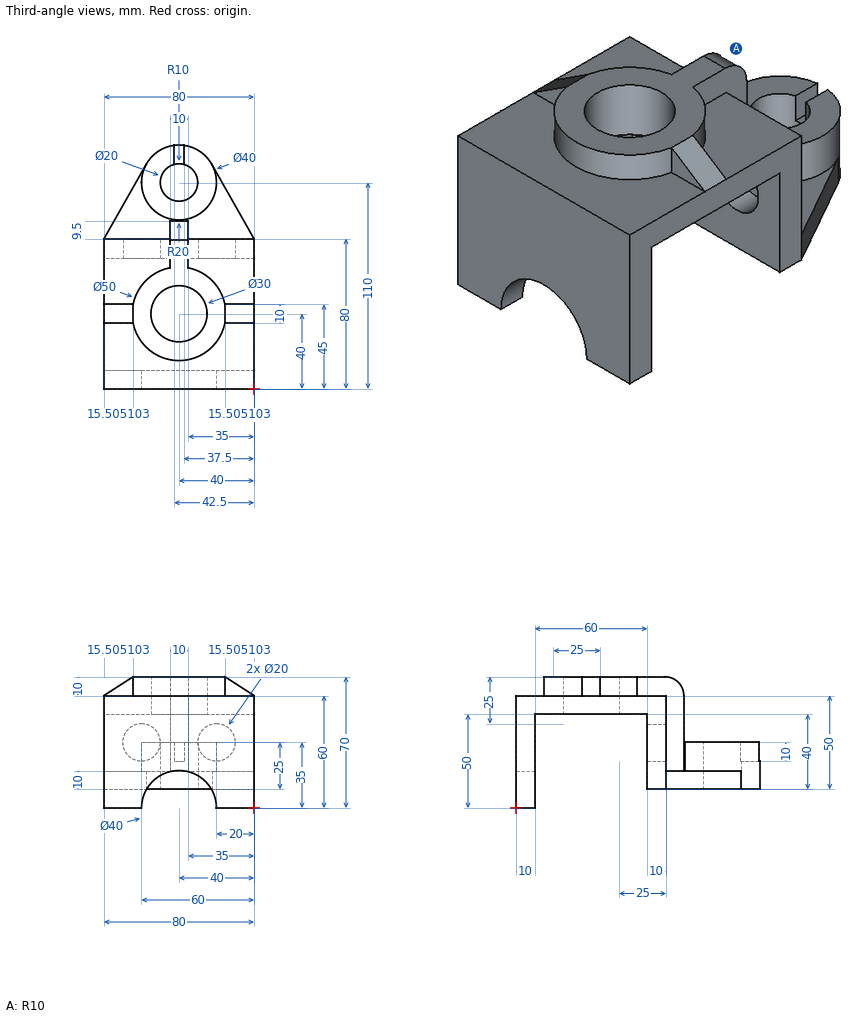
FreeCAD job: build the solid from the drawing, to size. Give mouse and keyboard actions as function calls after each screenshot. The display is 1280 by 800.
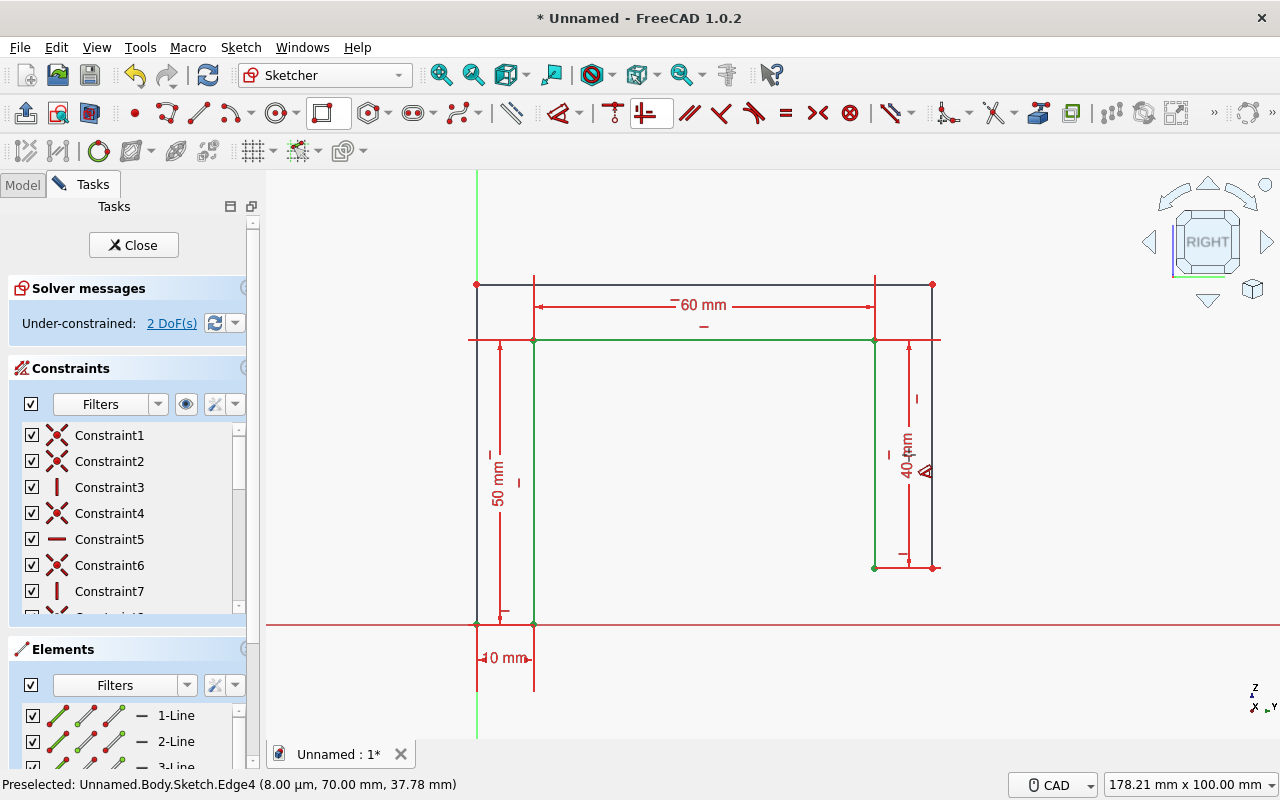
click(892, 568)
click(903, 602)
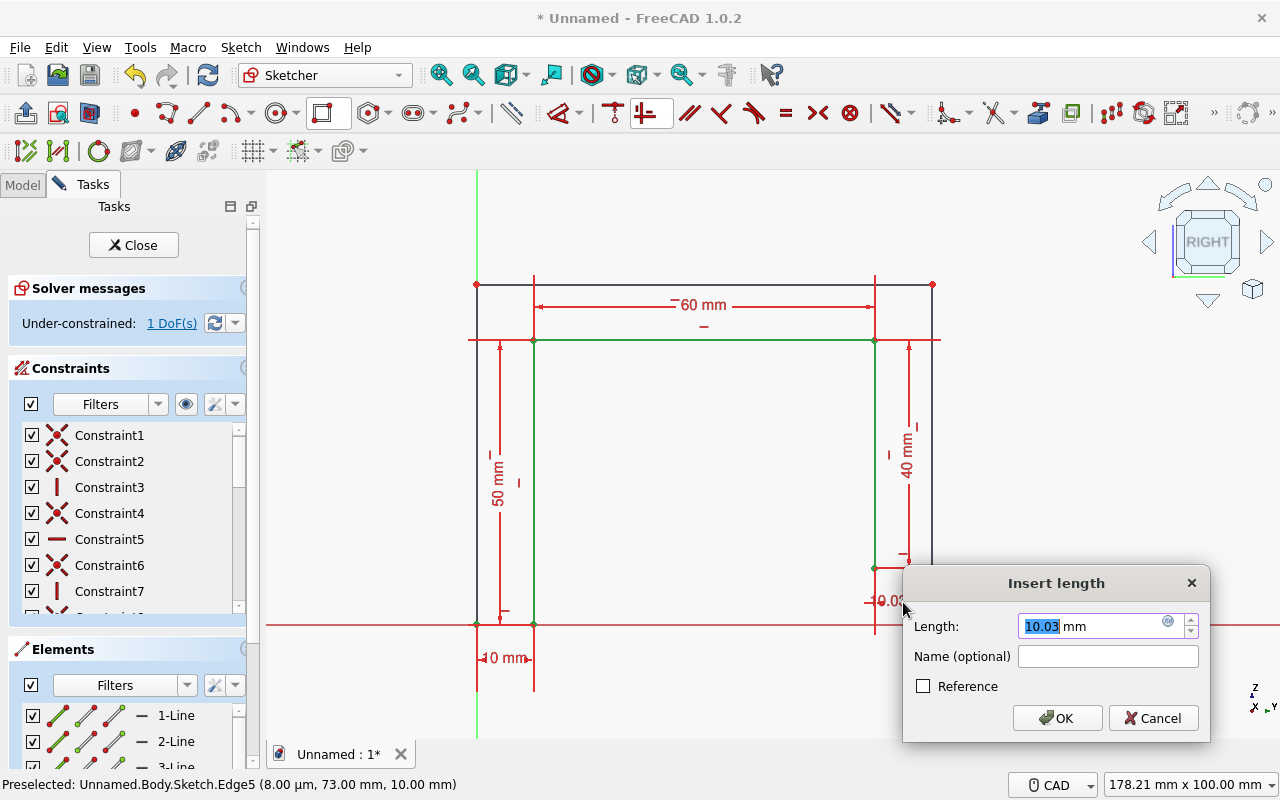
text(10)
key(Return)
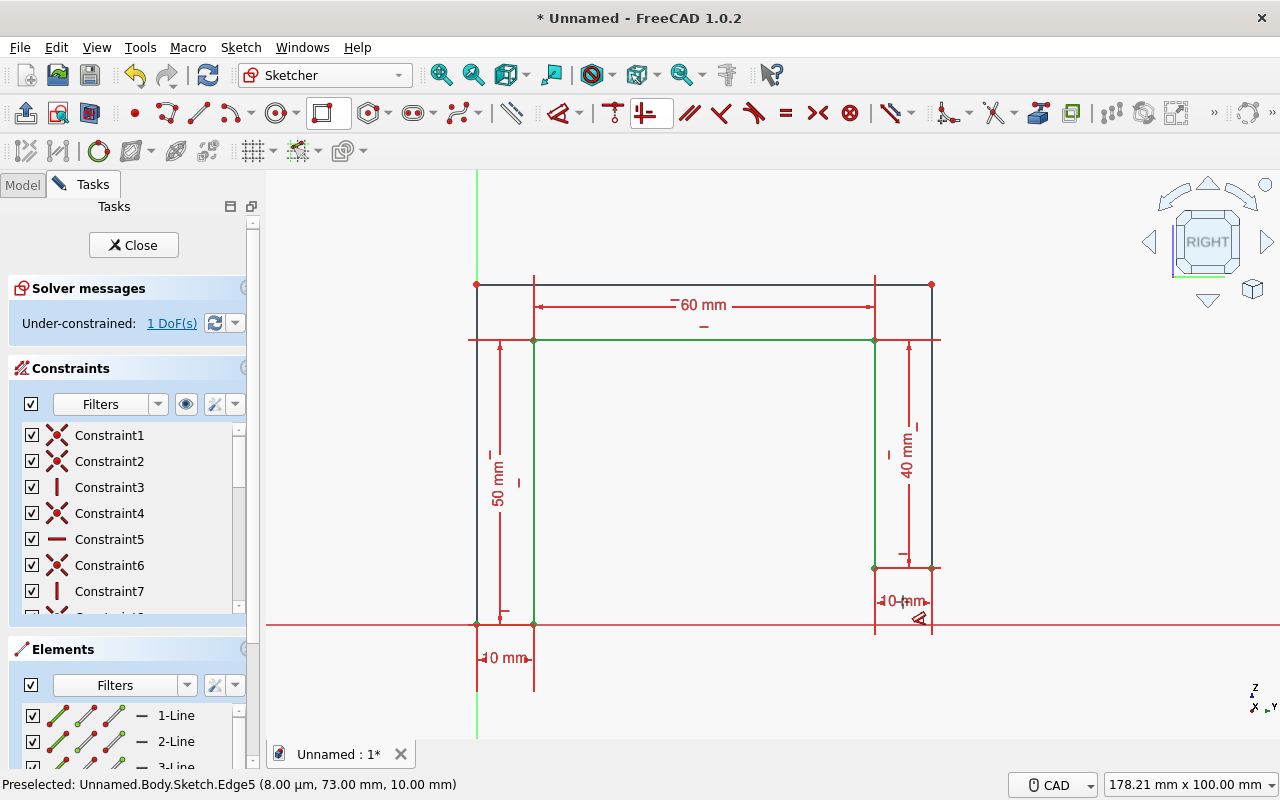
click(932, 483)
click(966, 427)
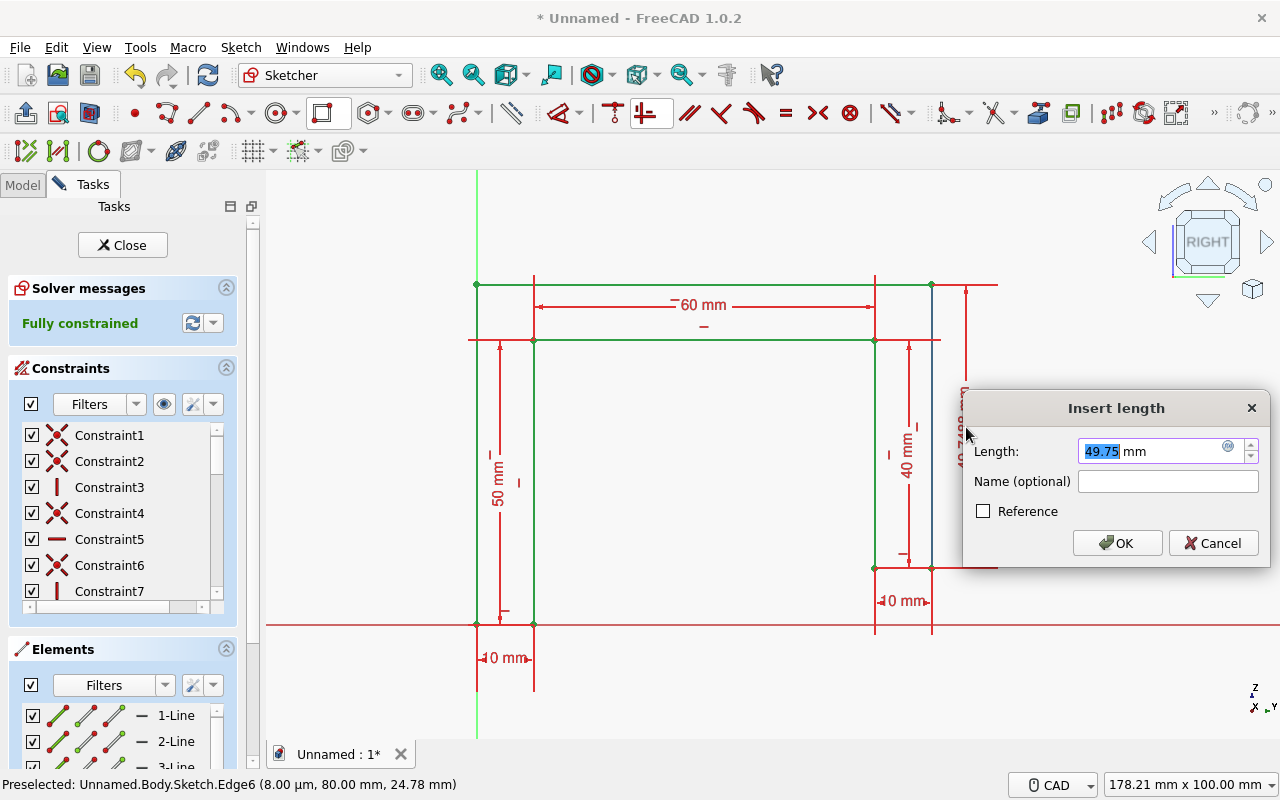
text(50)
key(Return)
key(Escape)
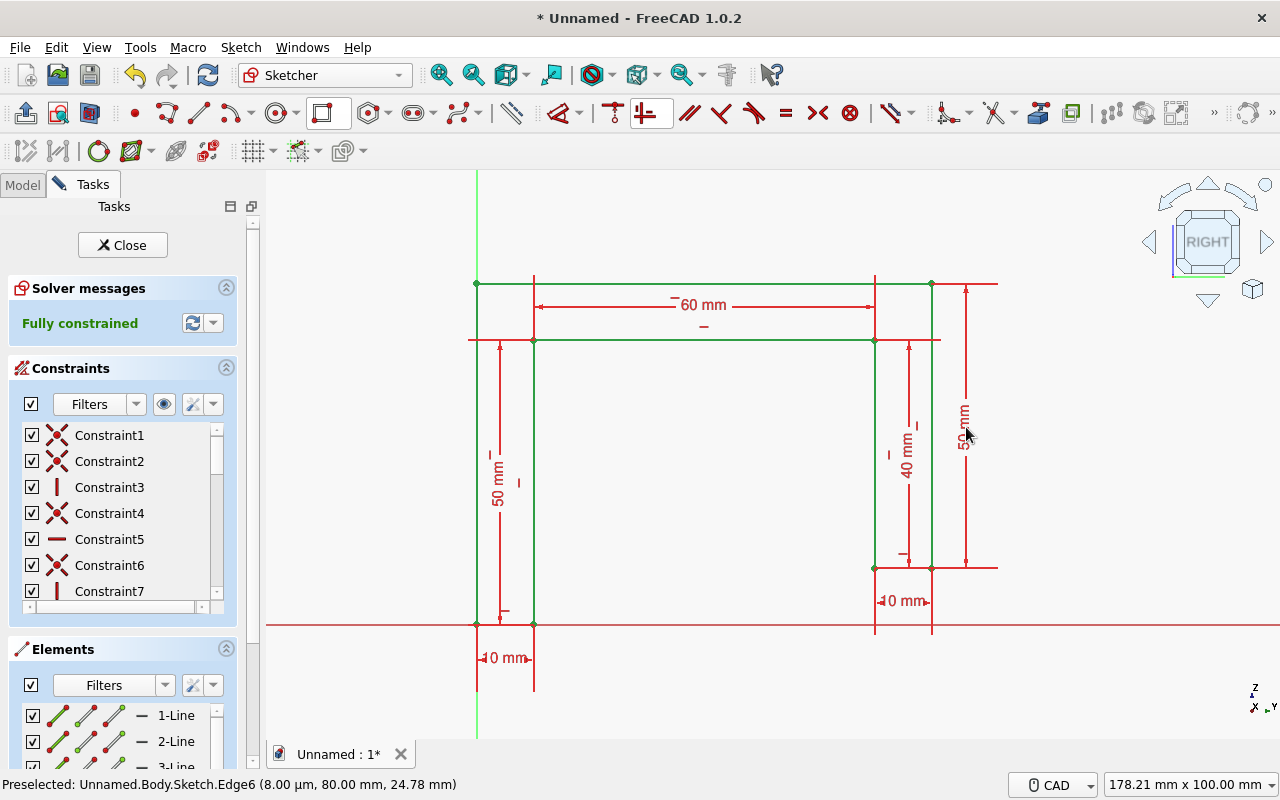
click(123, 245)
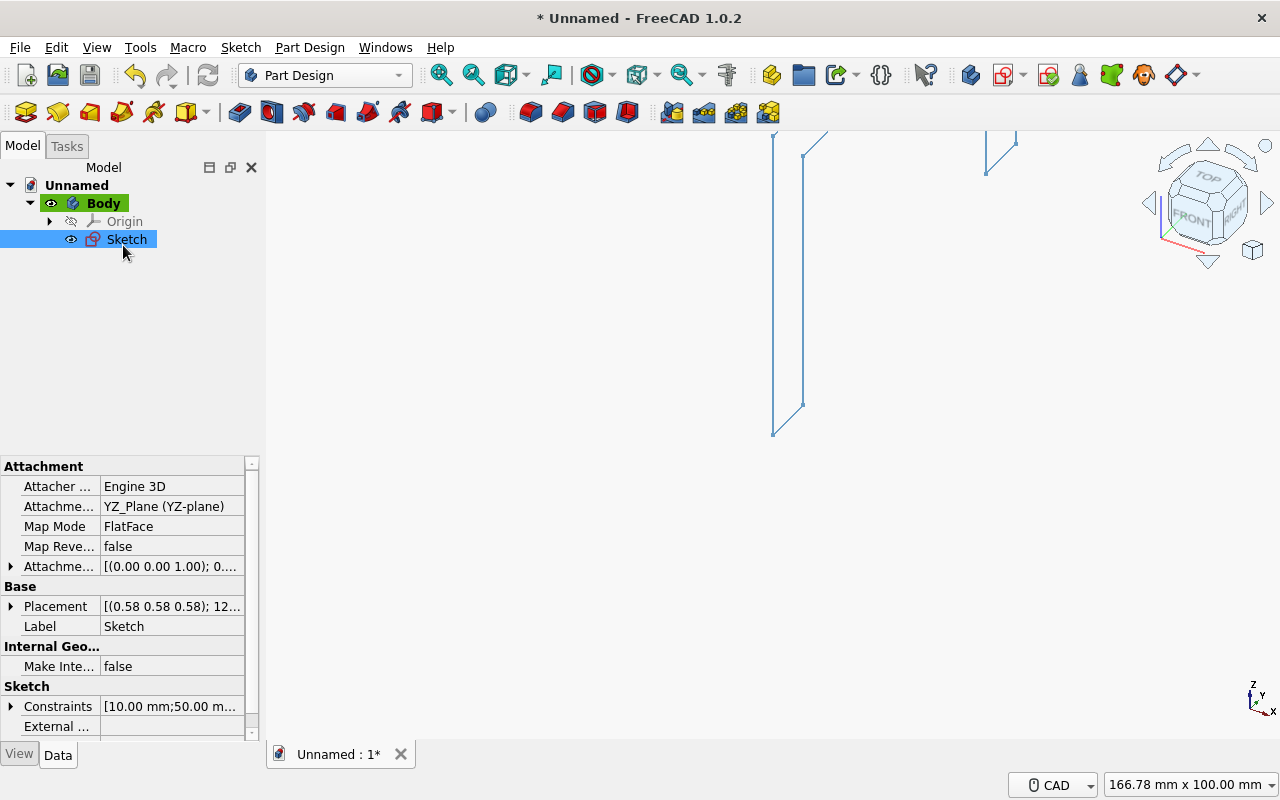
click(26, 112)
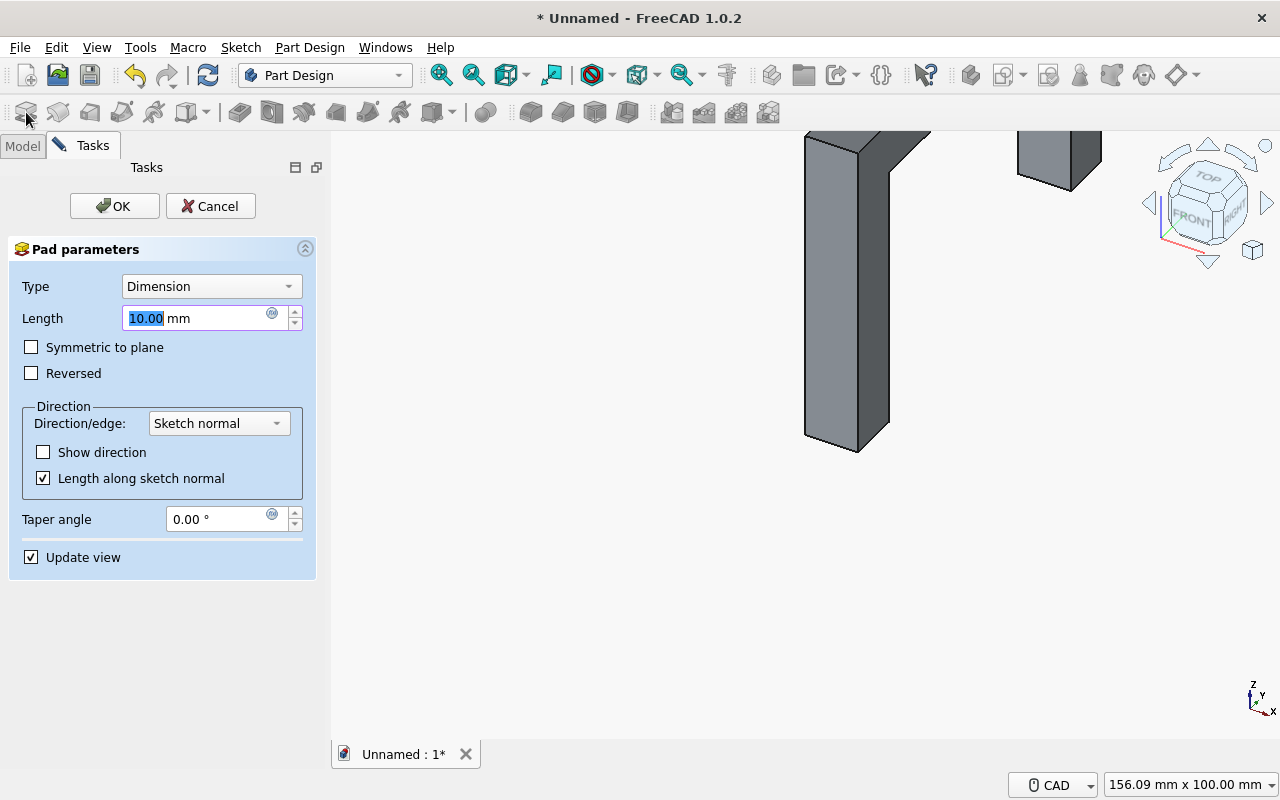
text(80)
key(Tab)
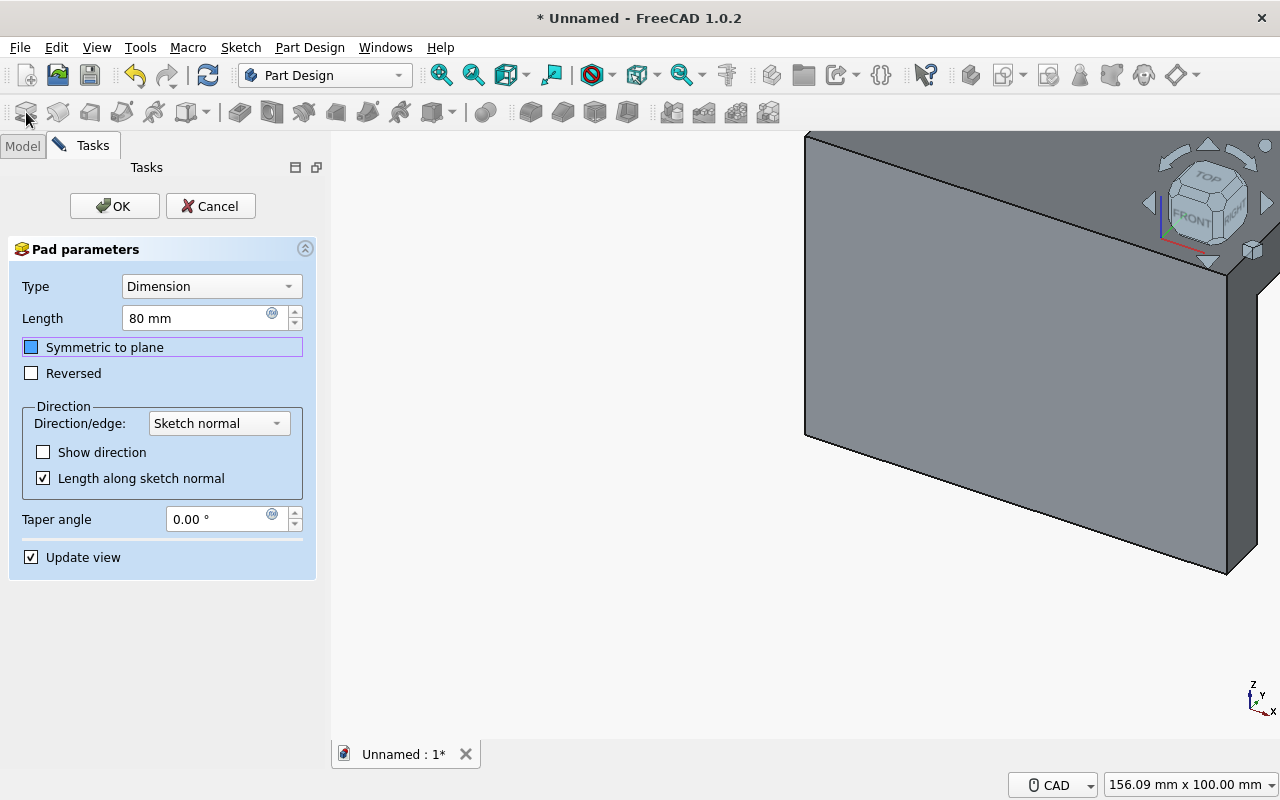
click(30, 373)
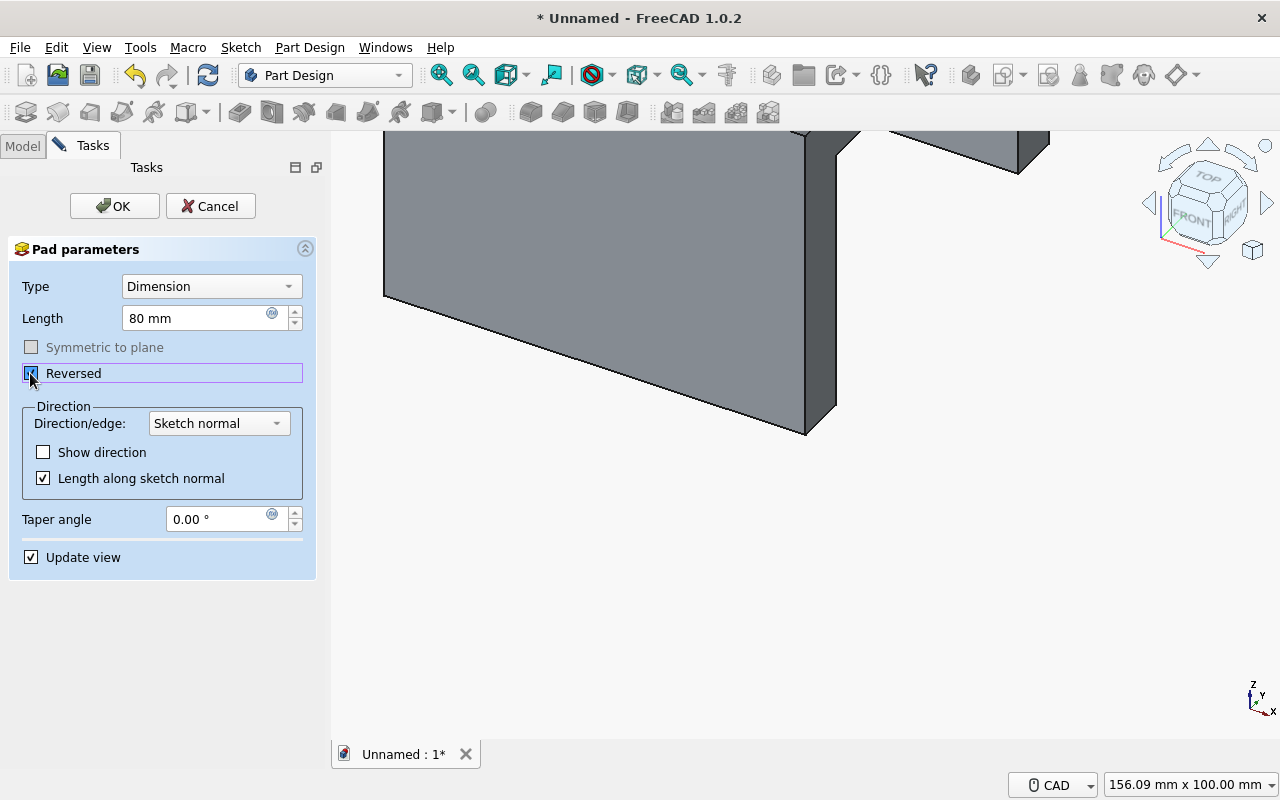
click(115, 206)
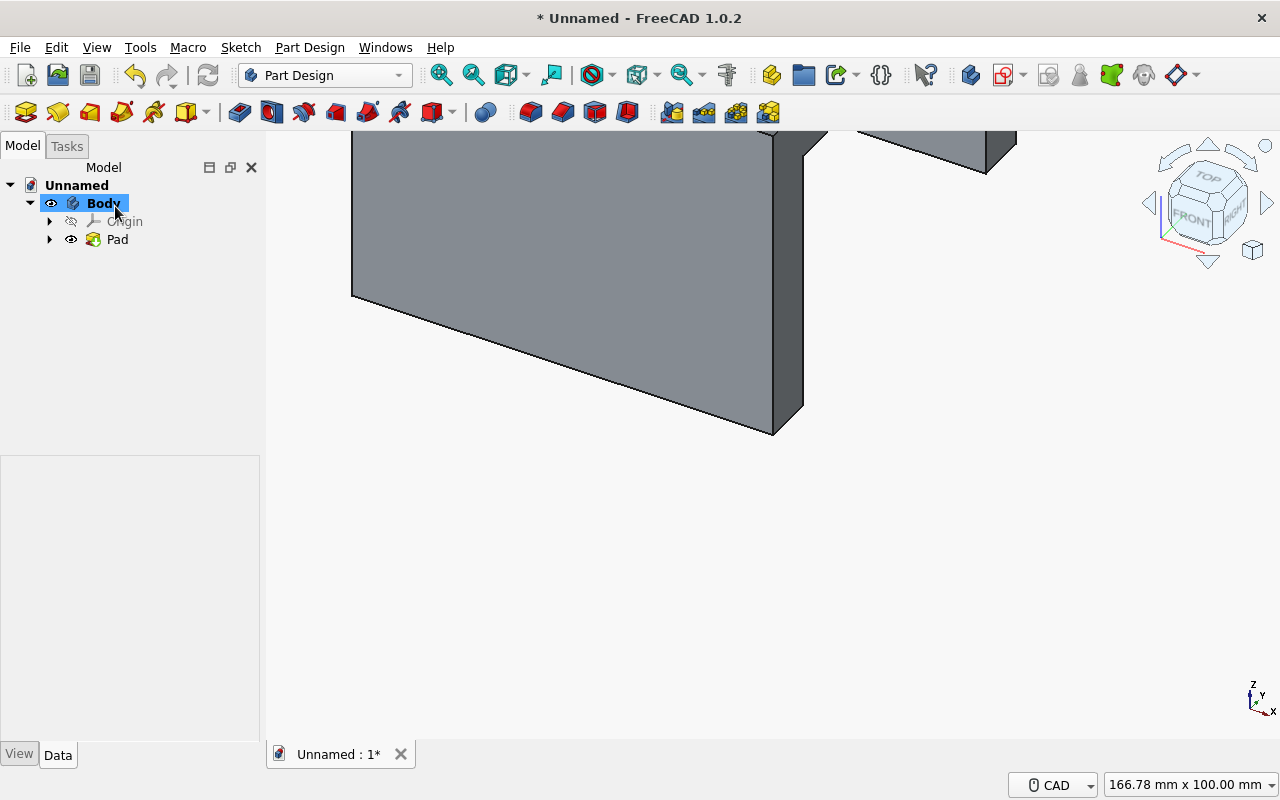
click(442, 76)